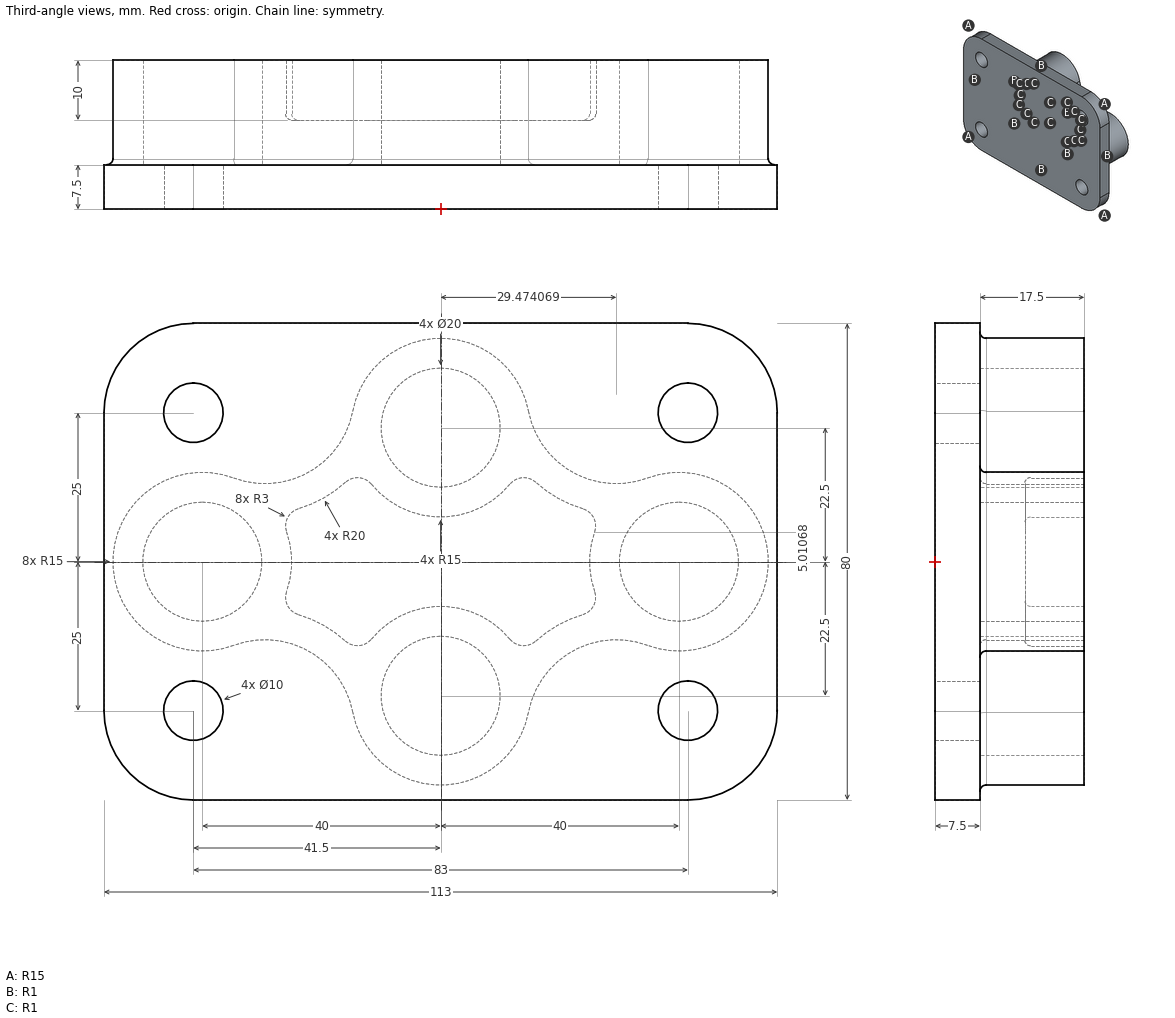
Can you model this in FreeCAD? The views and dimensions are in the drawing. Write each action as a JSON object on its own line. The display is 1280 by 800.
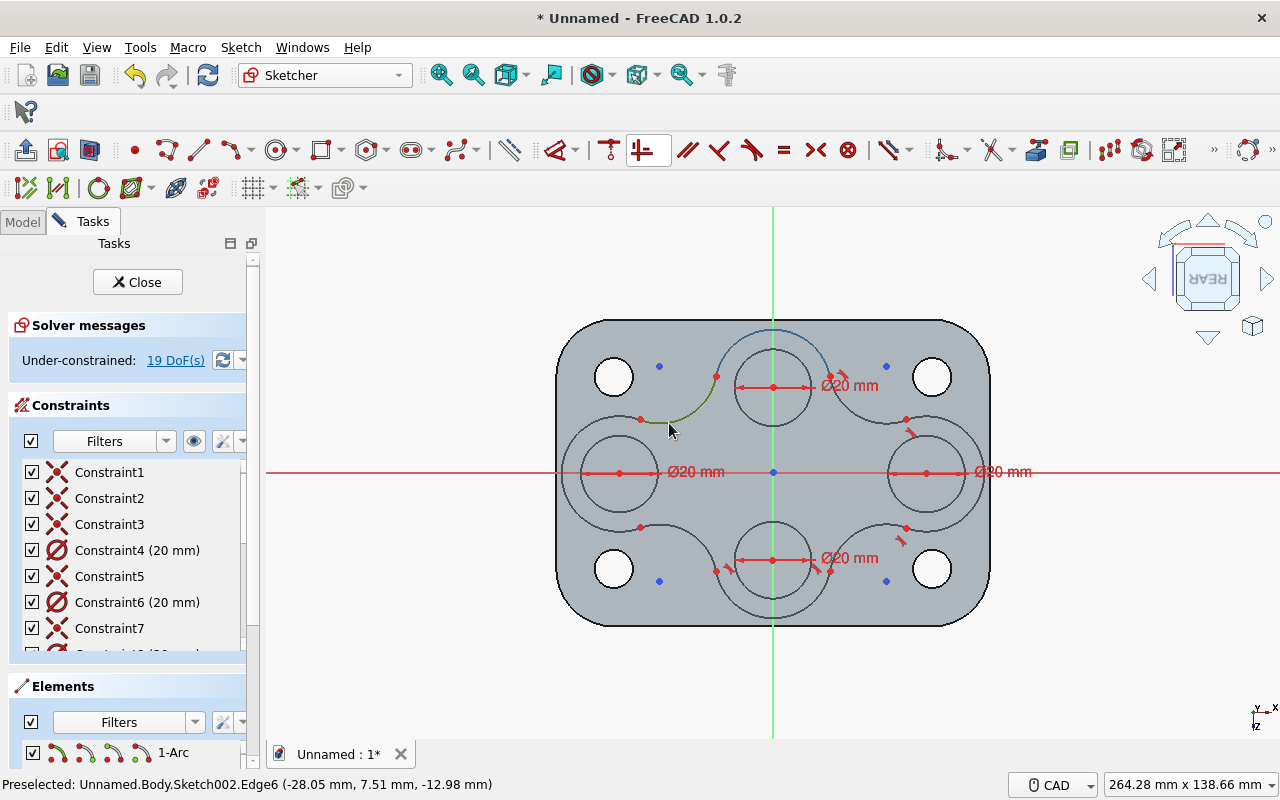
{"action": "key", "text": "t"}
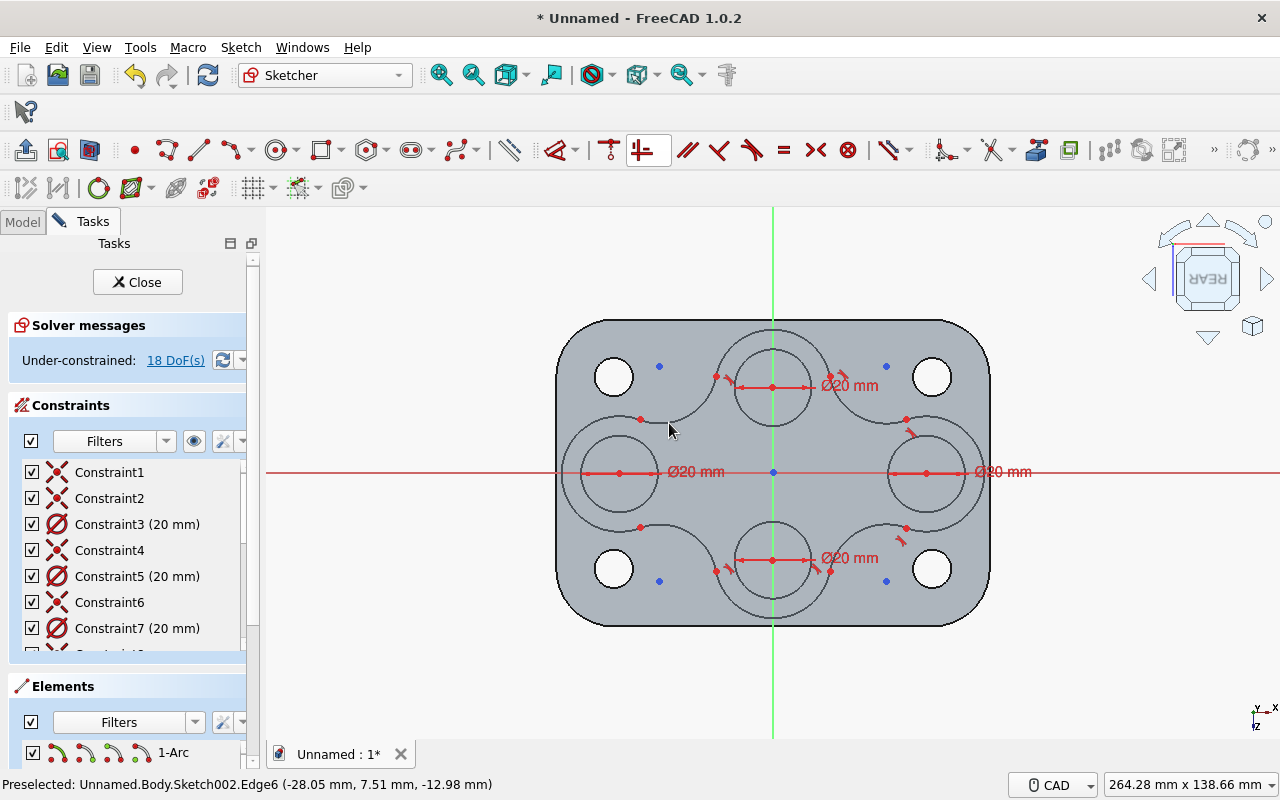
{"action": "left_click", "coordinate": [669, 423]}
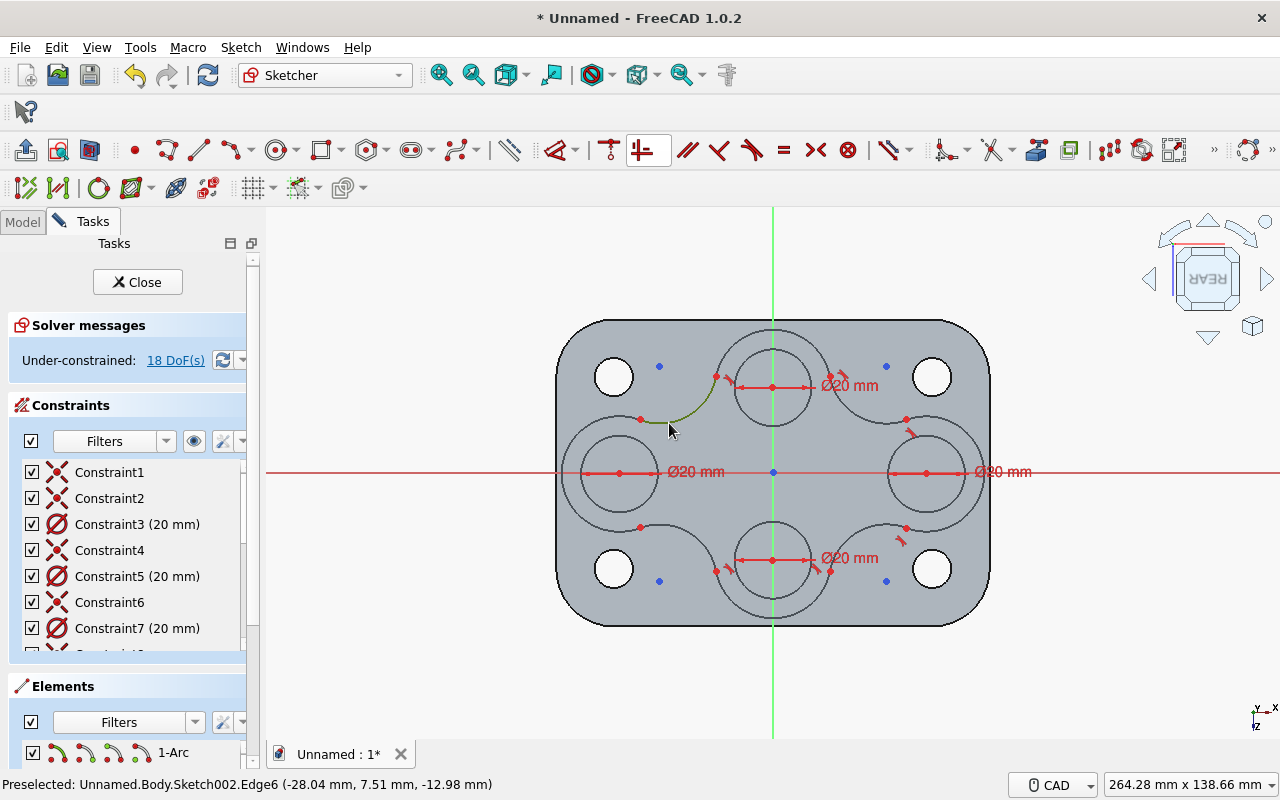
{"action": "left_click", "coordinate": [578, 434]}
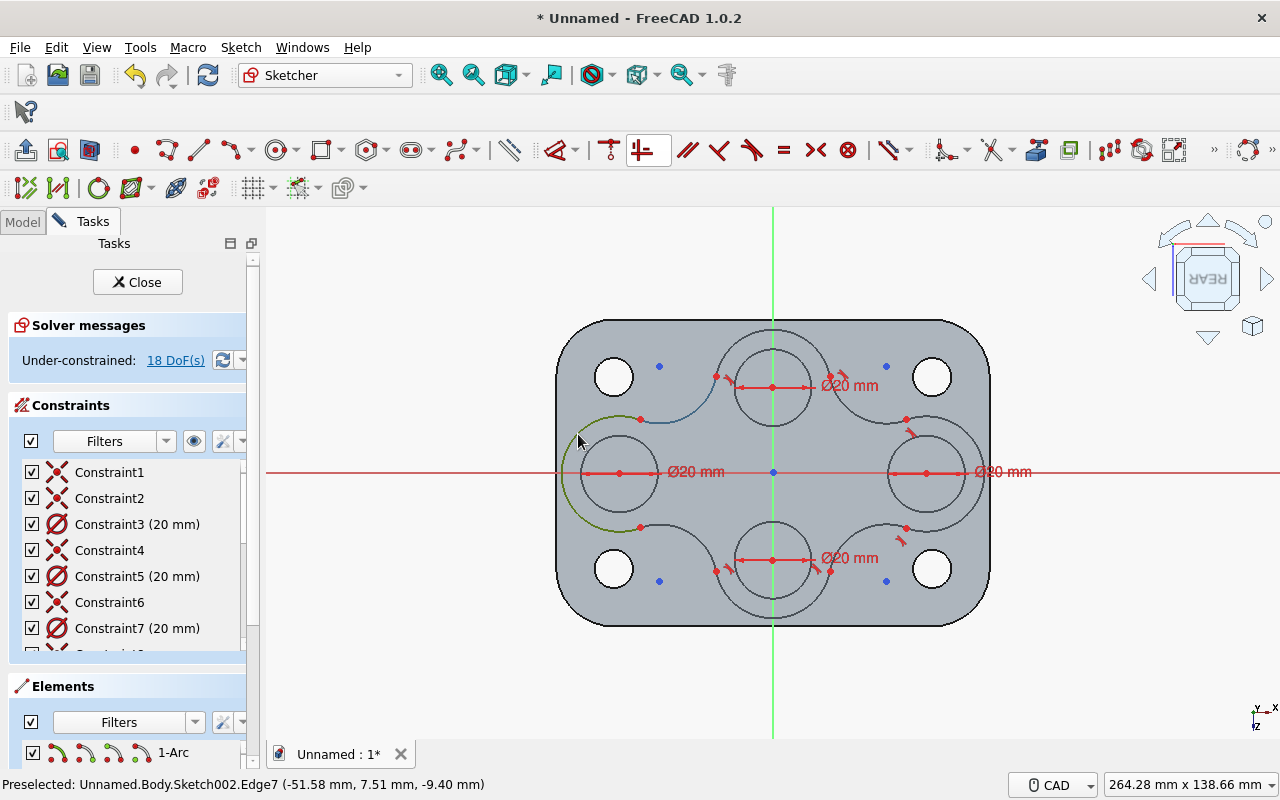
{"action": "left_click", "coordinate": [752, 150]}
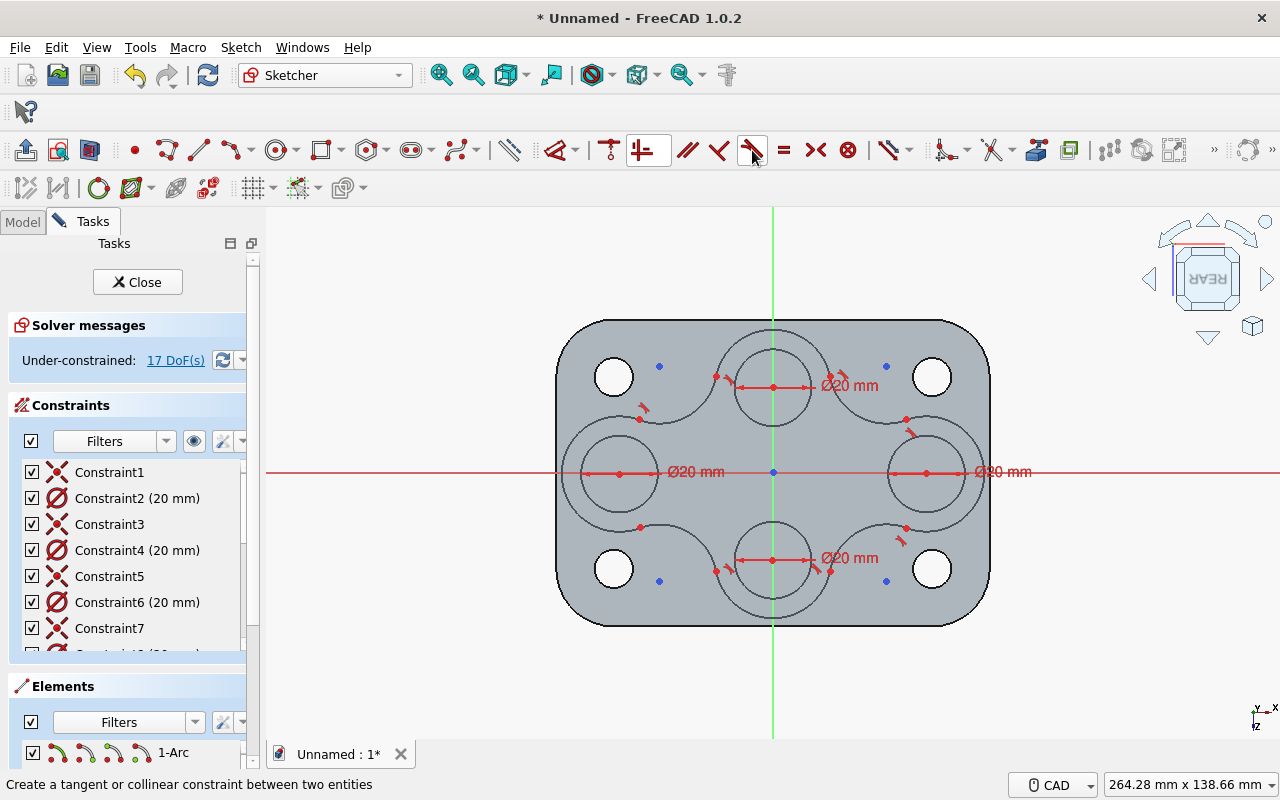
{"action": "left_click", "coordinate": [578, 434]}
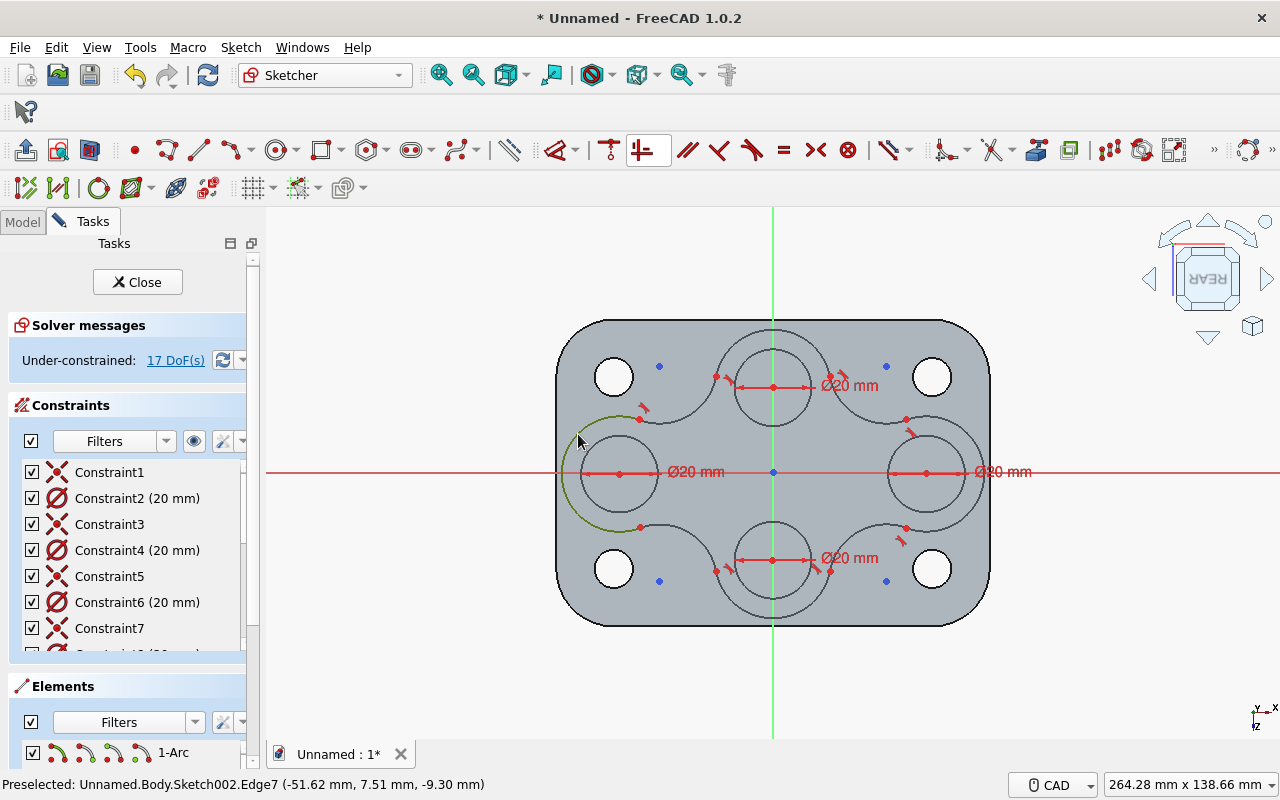
{"action": "left_click", "coordinate": [703, 545]}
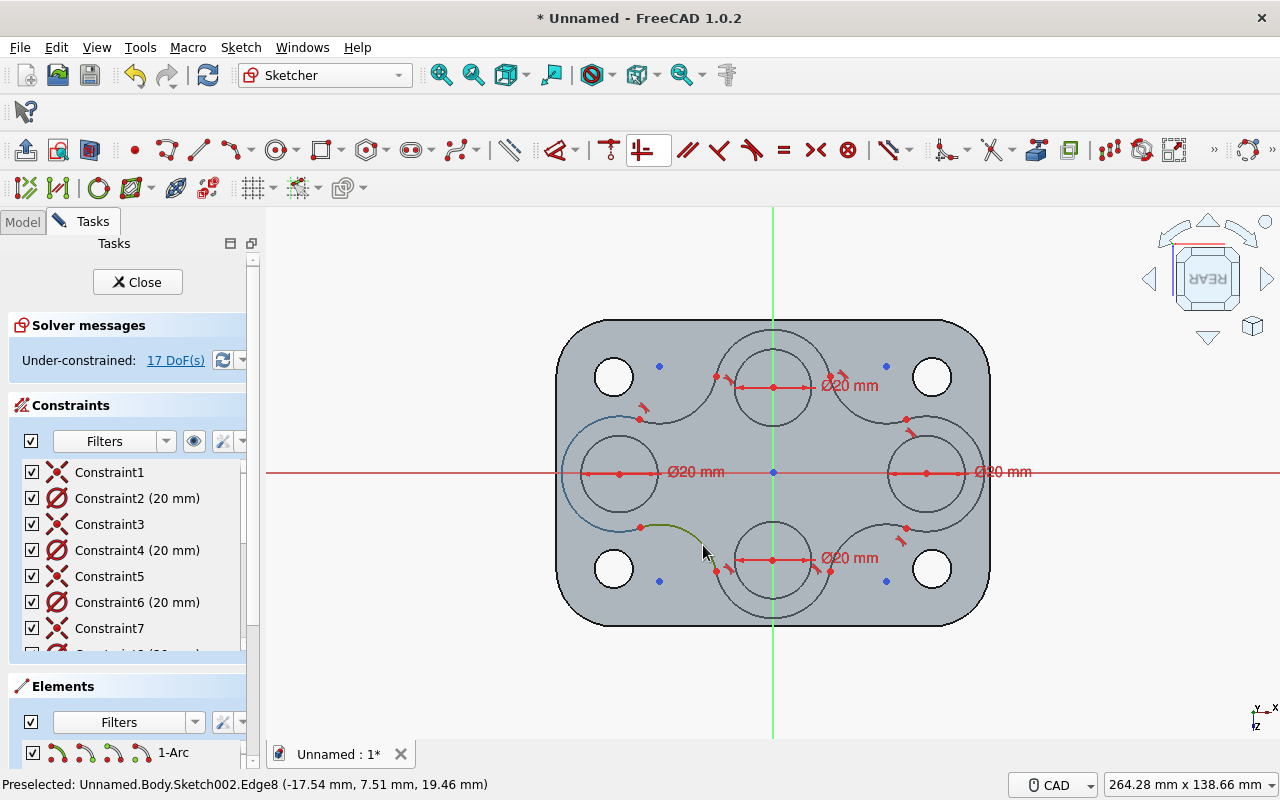
{"action": "key", "text": "t"}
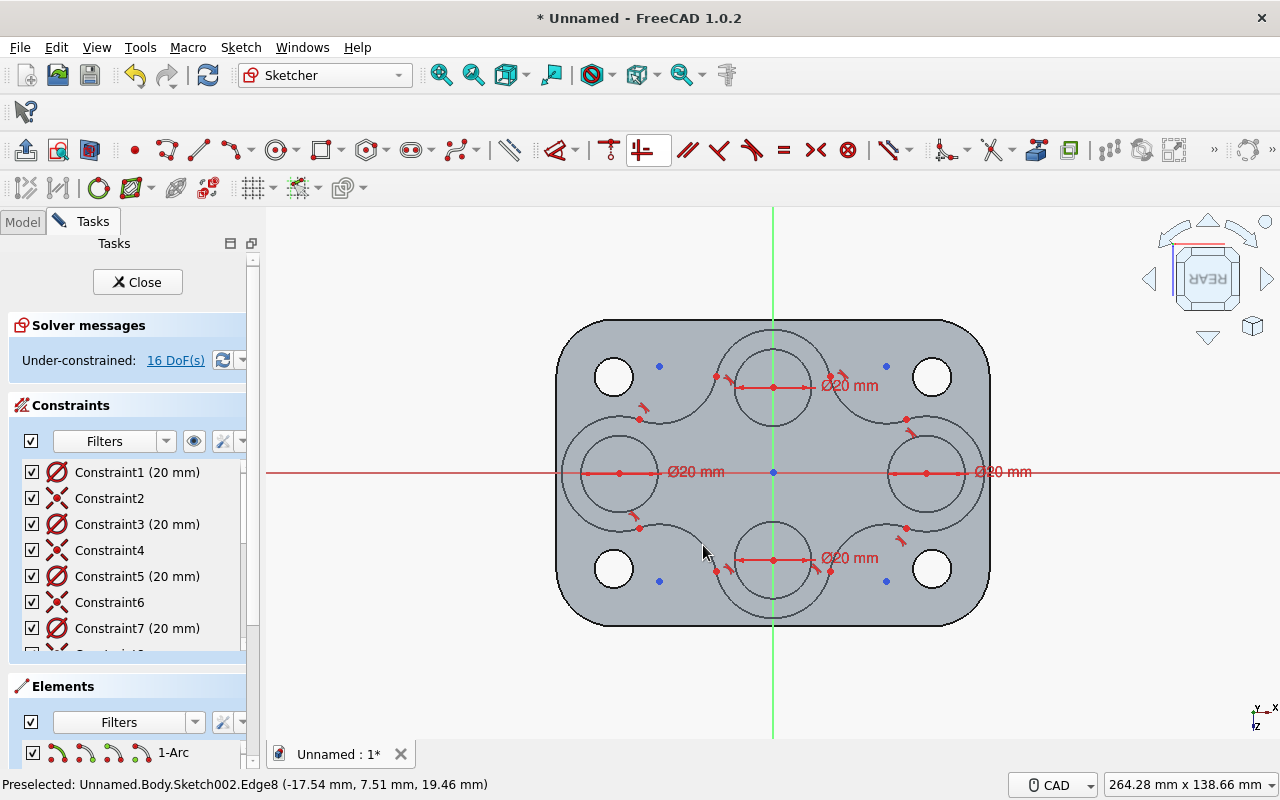
{"action": "left_click", "coordinate": [743, 610]}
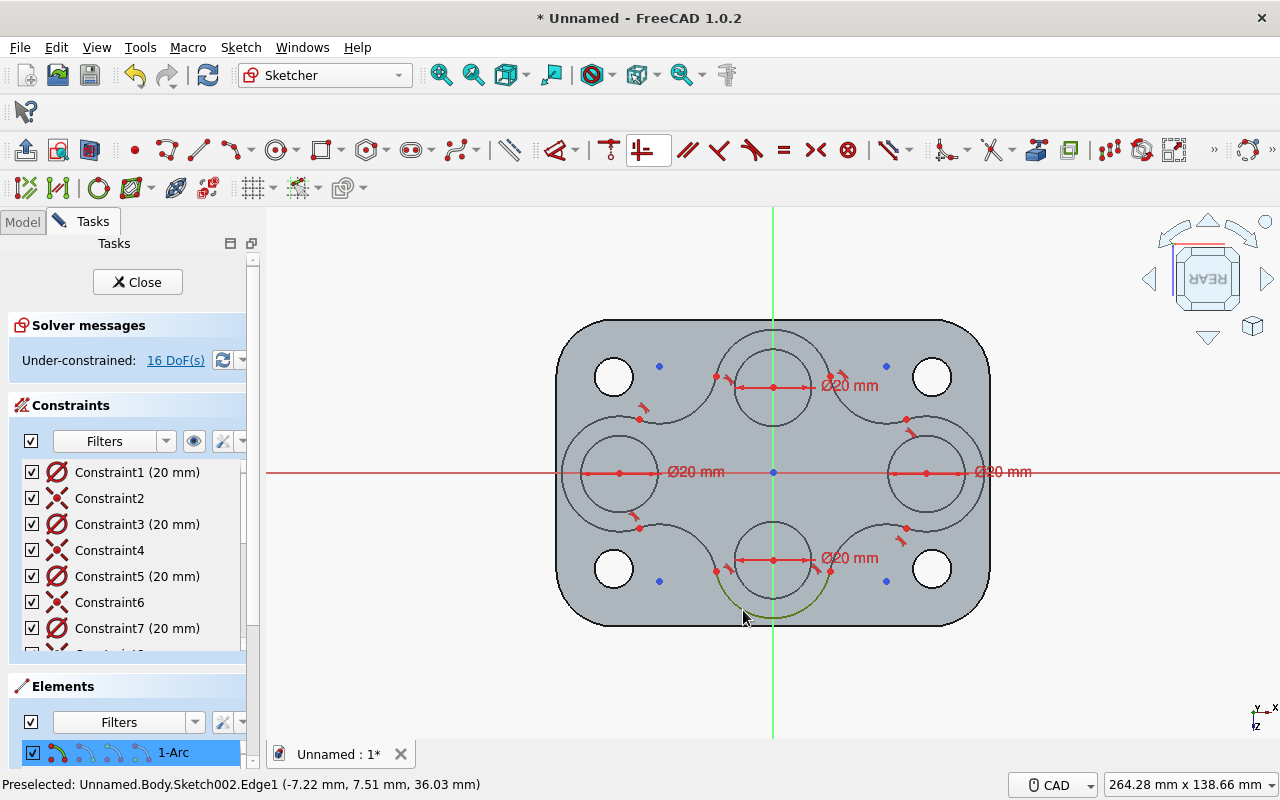
{"action": "left_click", "coordinate": [877, 525]}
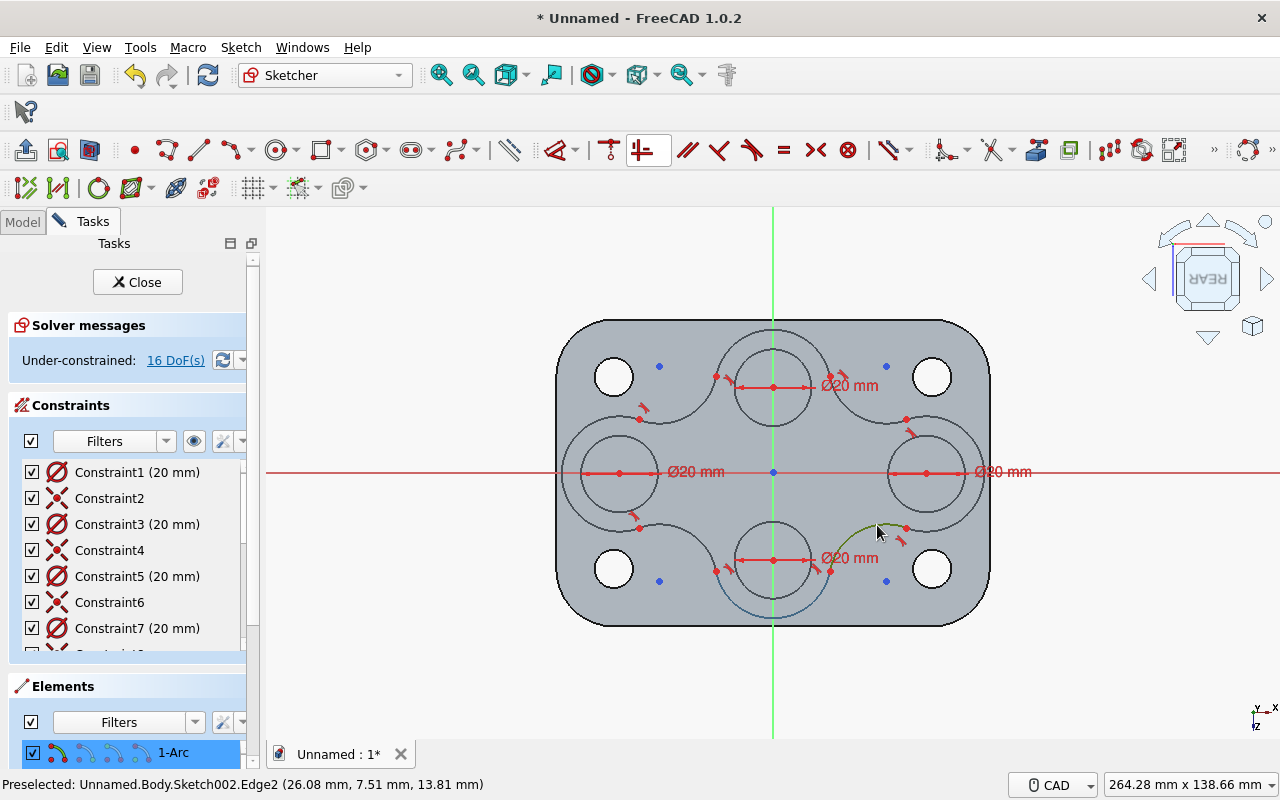
{"action": "left_click", "coordinate": [968, 514]}